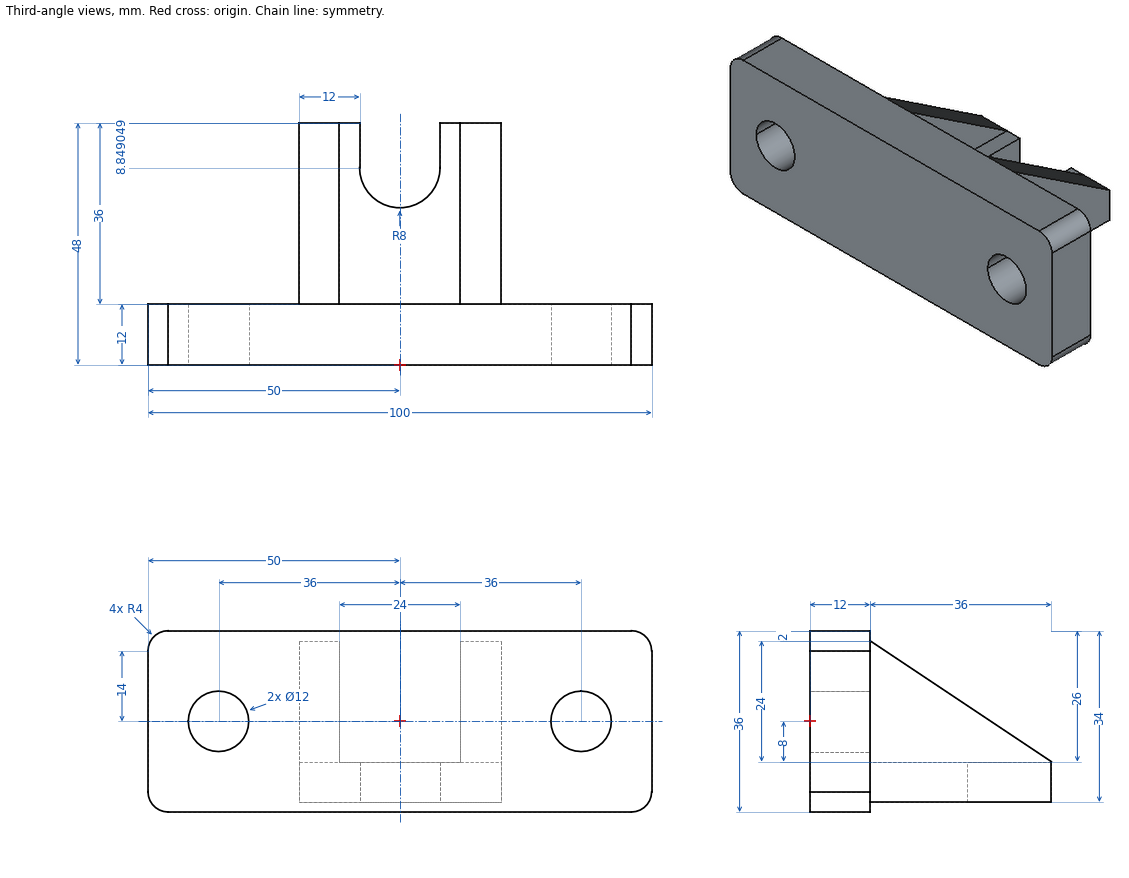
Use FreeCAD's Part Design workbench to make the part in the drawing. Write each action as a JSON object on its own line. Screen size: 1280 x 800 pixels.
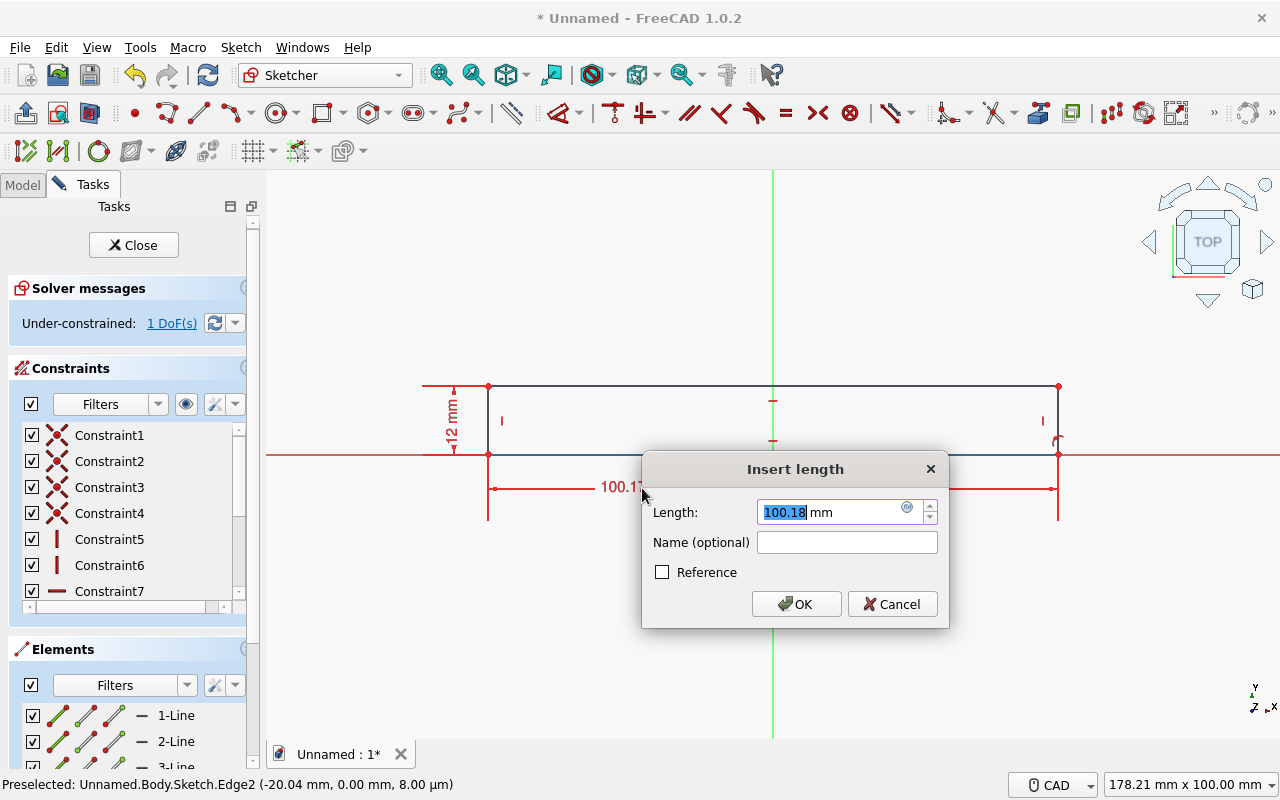
{"action": "type", "text": "100"}
{"action": "key", "text": "Return"}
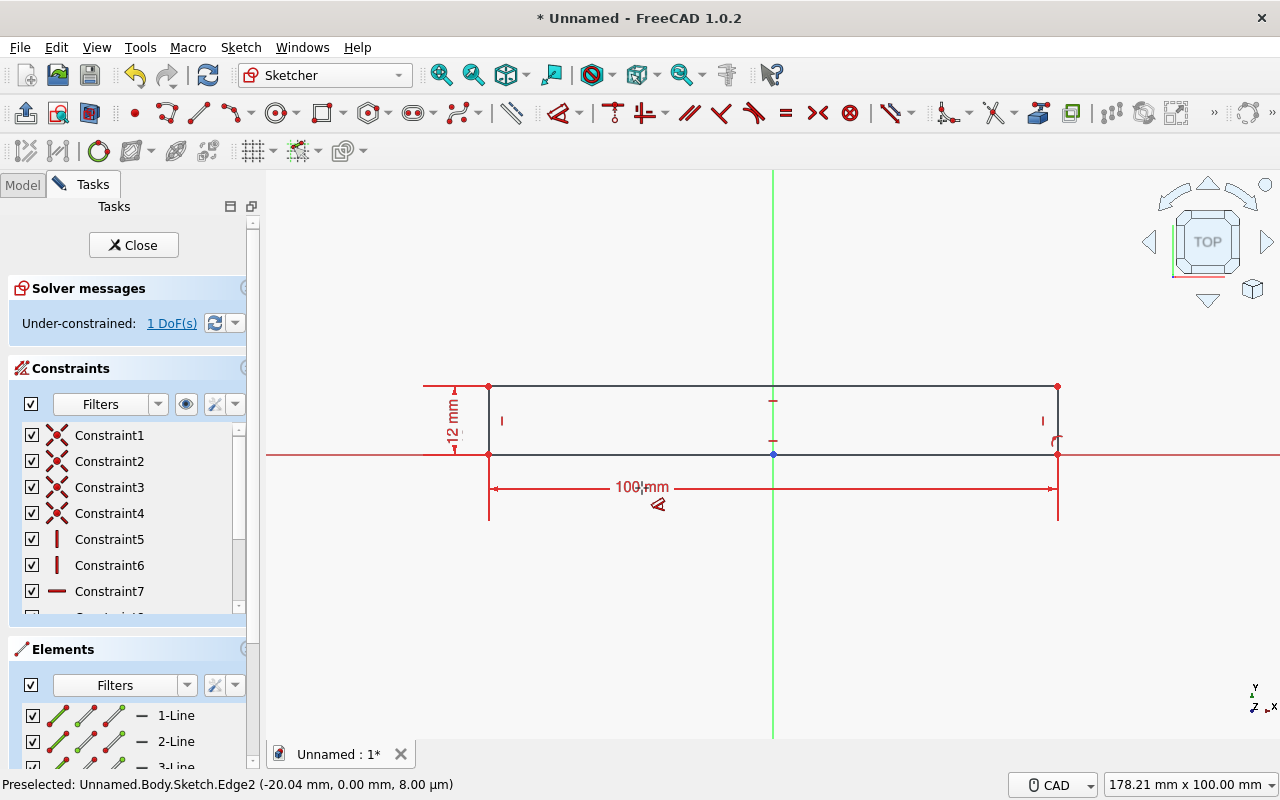
{"action": "left_click", "coordinate": [489, 386]}
{"action": "left_click", "coordinate": [565, 488]}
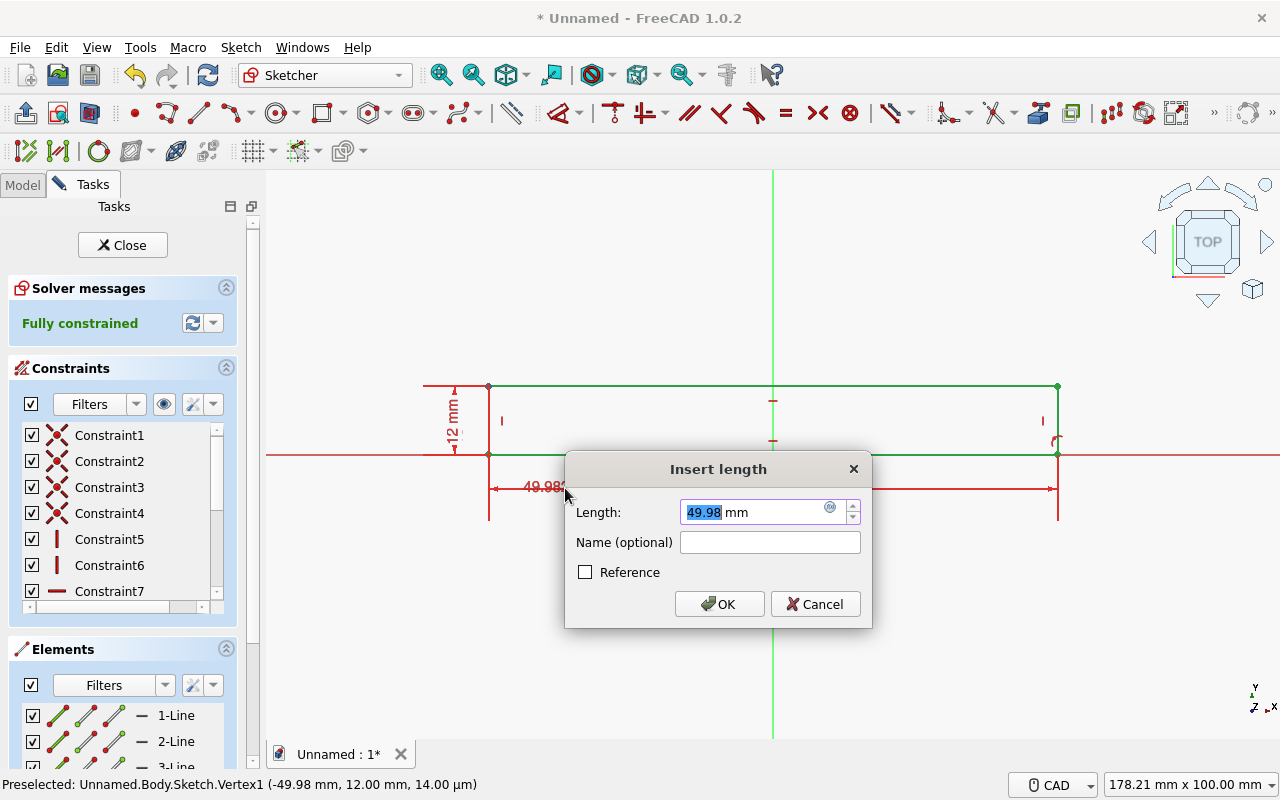
{"action": "type", "text": "50"}
{"action": "key", "text": "Return"}
{"action": "key", "text": "Escape"}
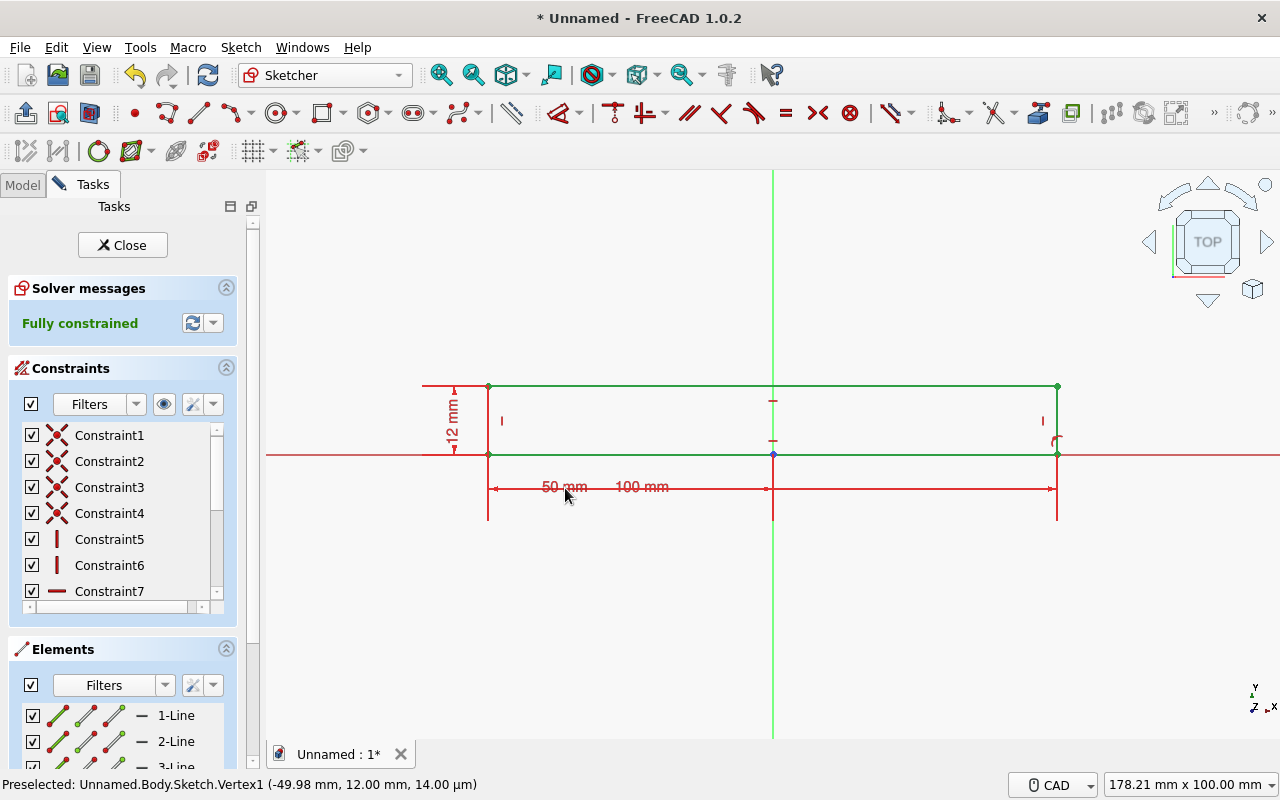
{"action": "left_click", "coordinate": [123, 245]}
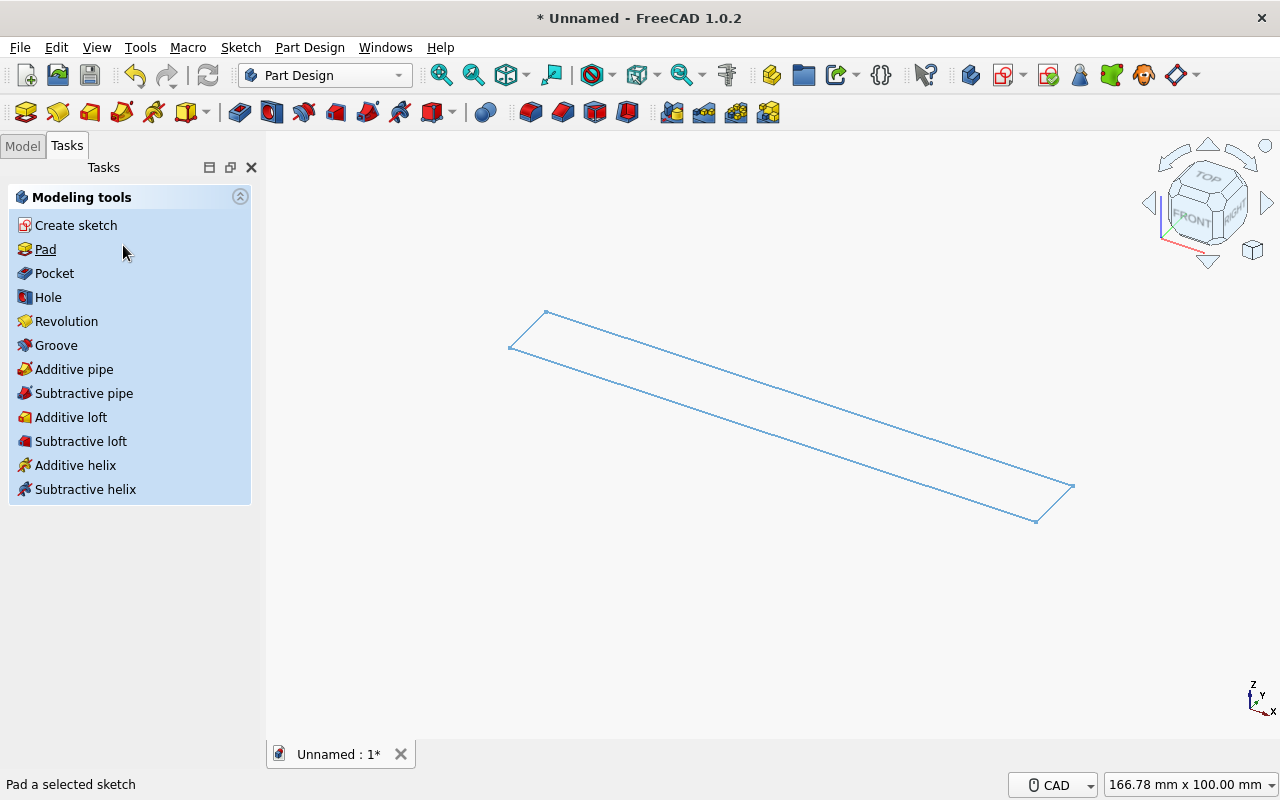
{"action": "left_click", "coordinate": [26, 112]}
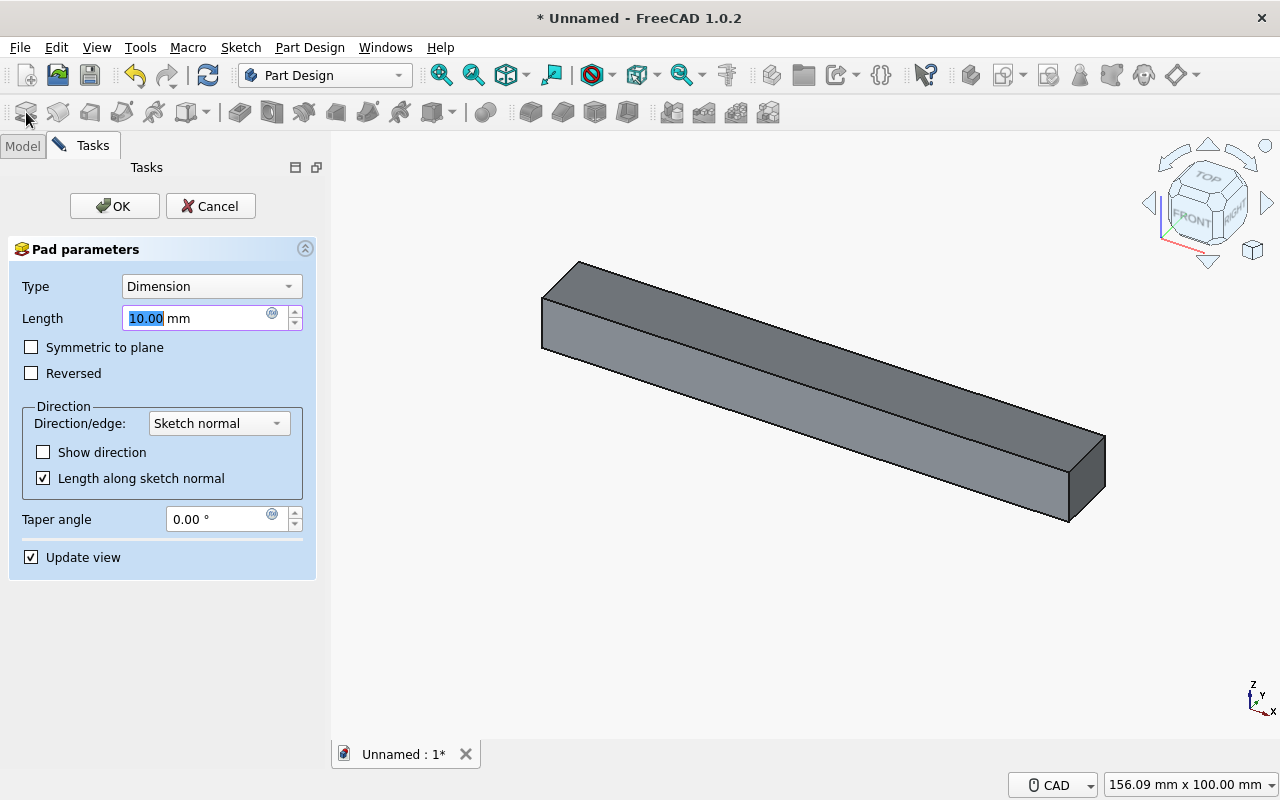
{"action": "type", "text": "36"}
{"action": "key", "text": "Tab"}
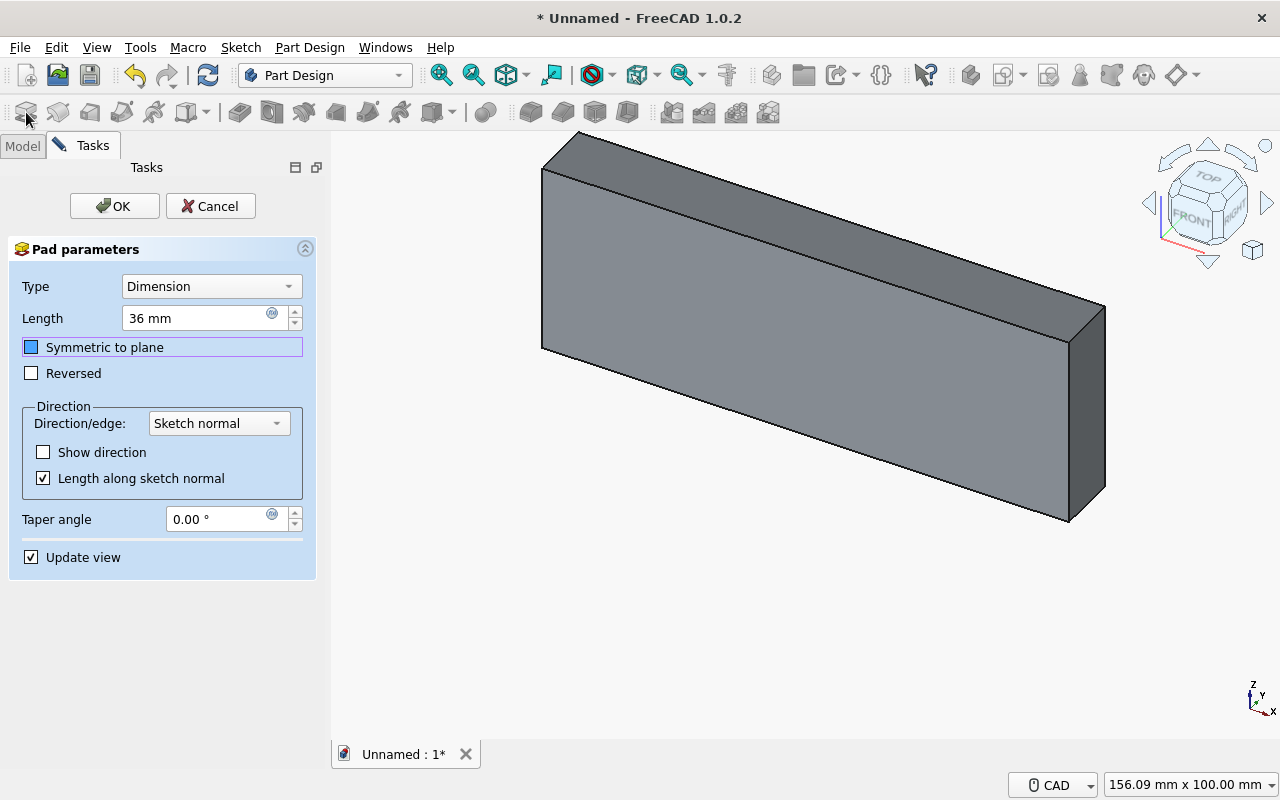
{"action": "left_click", "coordinate": [30, 347]}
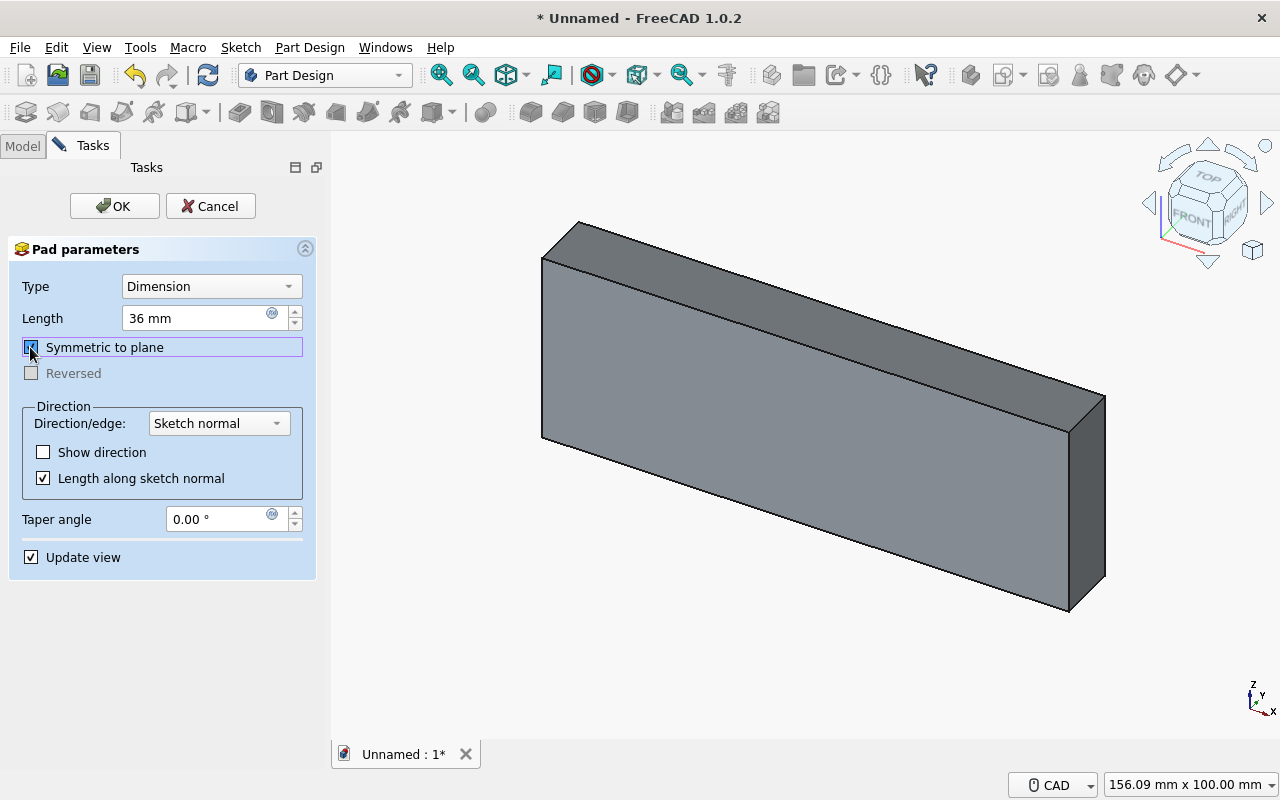
{"action": "left_click", "coordinate": [115, 206]}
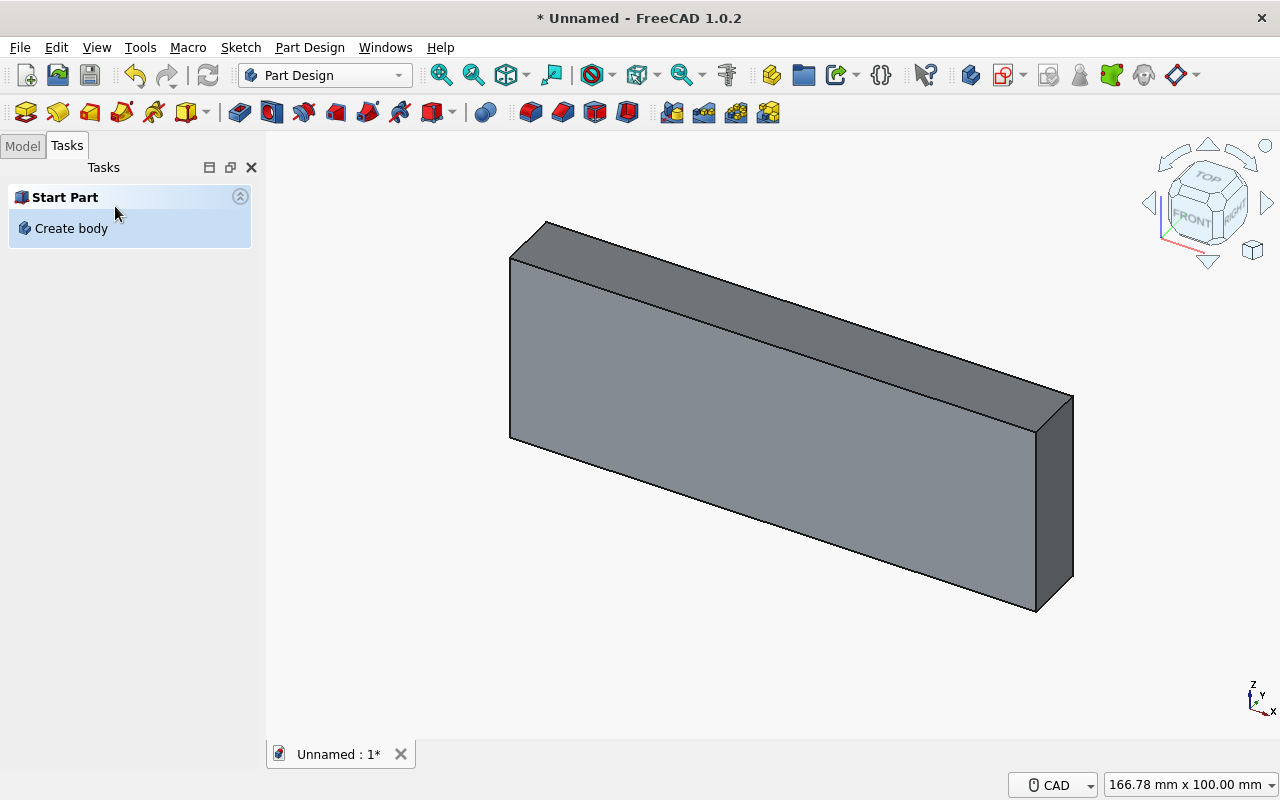
{"action": "key", "text": "4"}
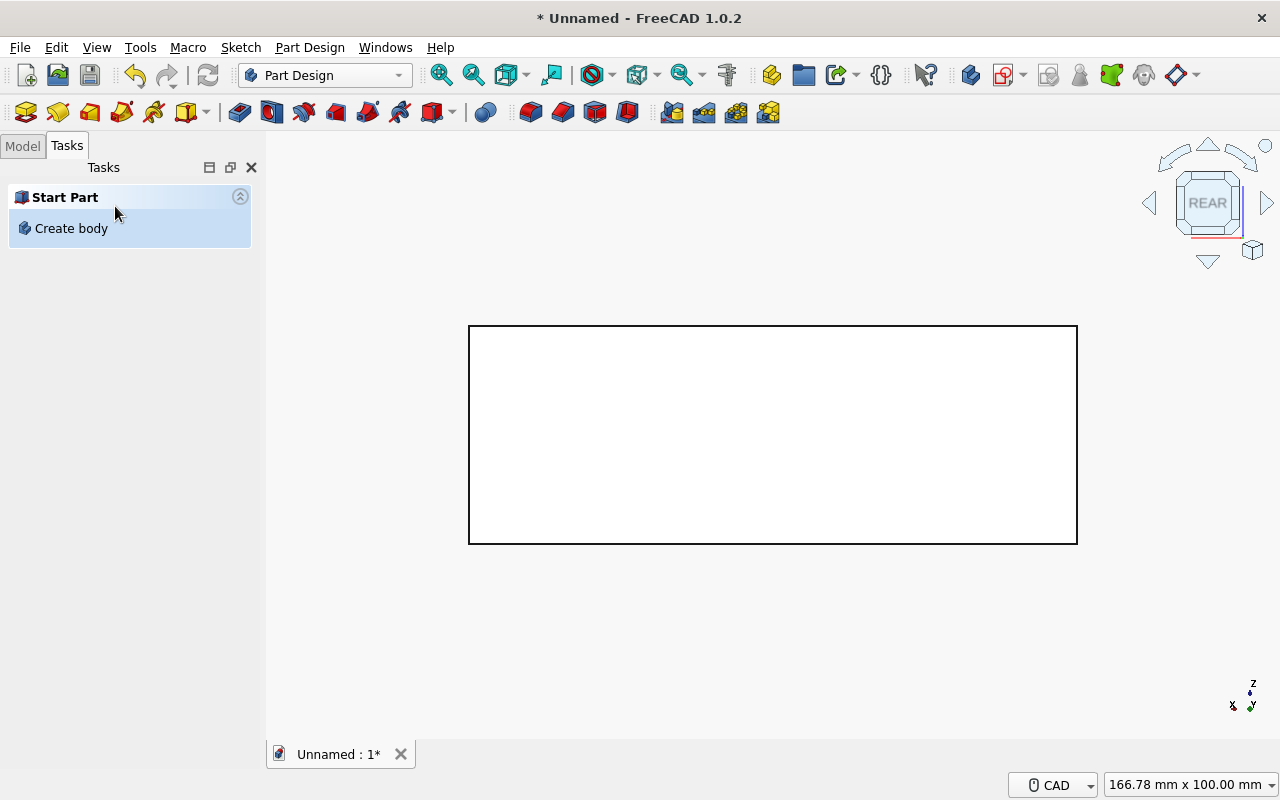
{"action": "left_click", "coordinate": [599, 434]}